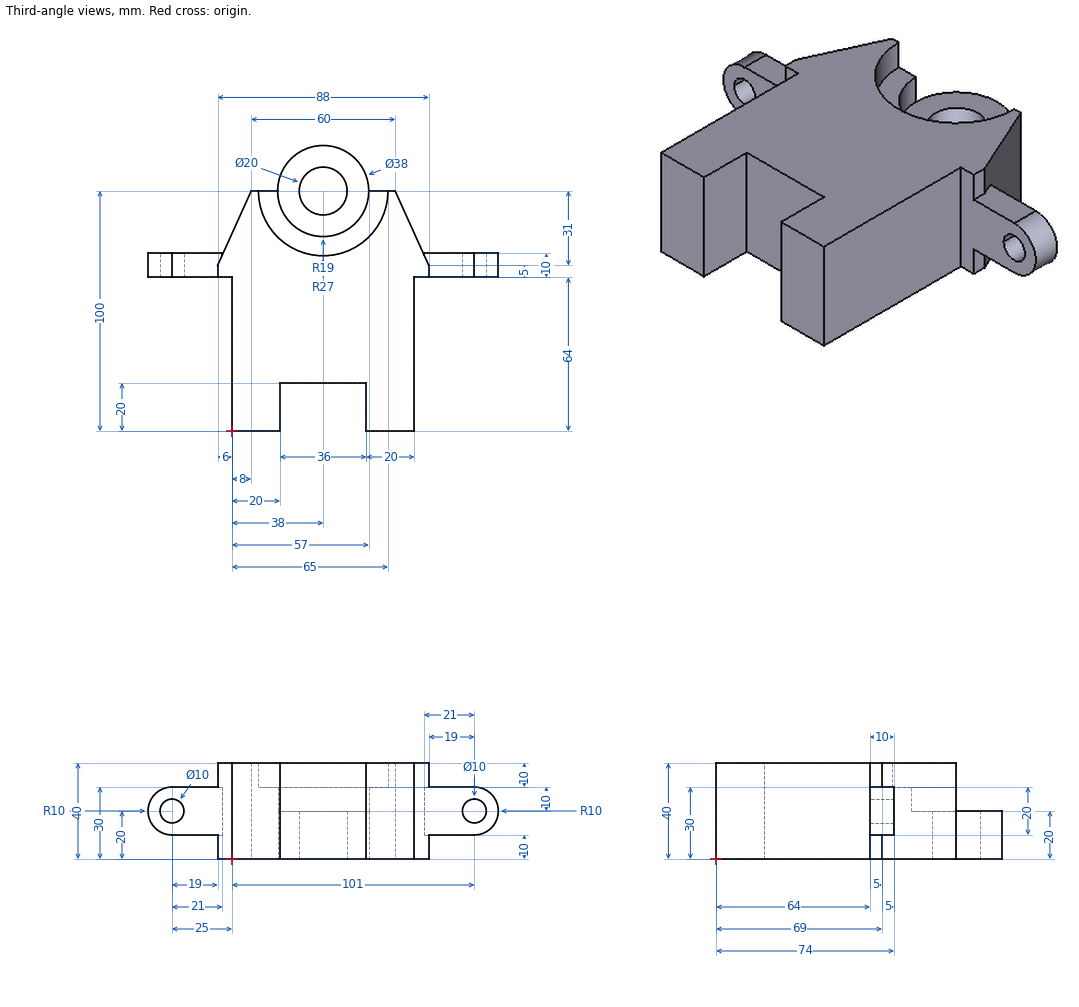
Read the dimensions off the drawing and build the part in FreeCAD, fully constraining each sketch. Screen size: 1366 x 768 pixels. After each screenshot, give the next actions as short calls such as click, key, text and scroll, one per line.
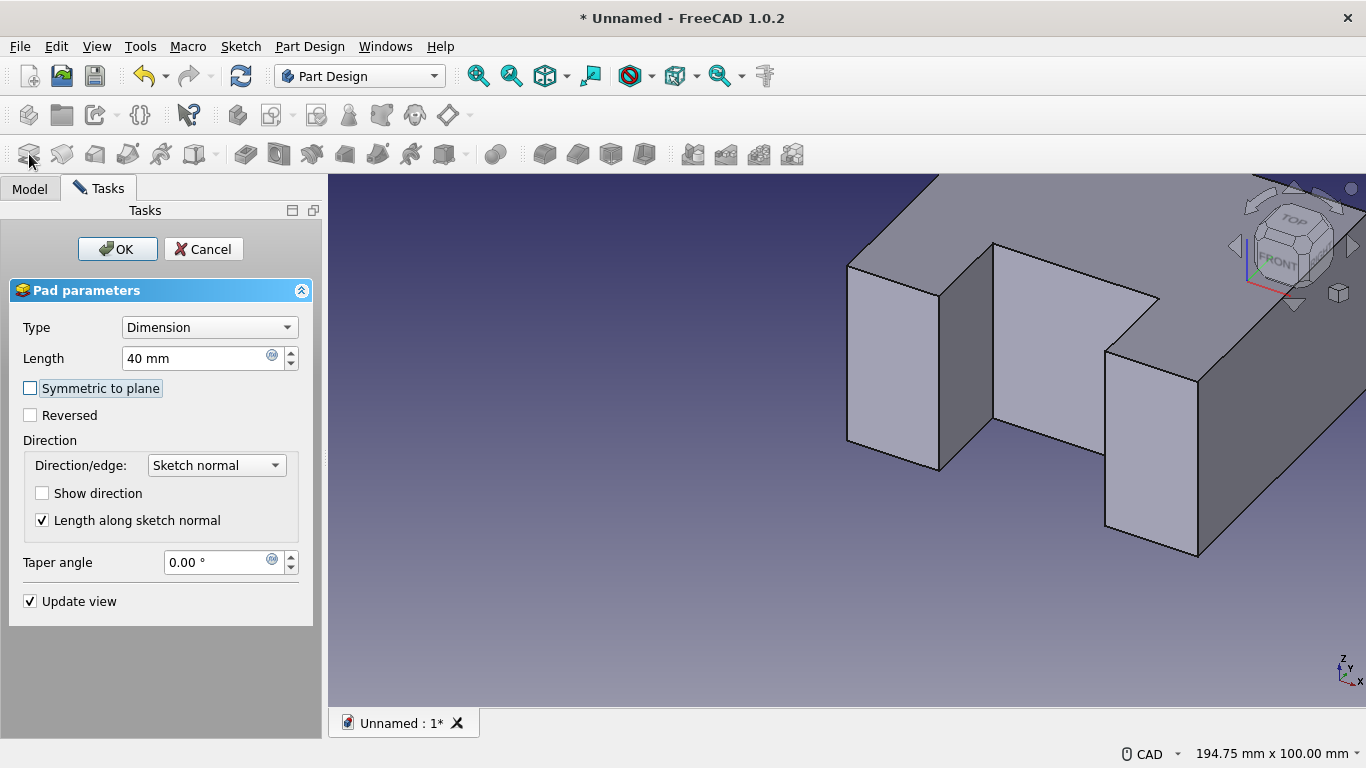
click(118, 249)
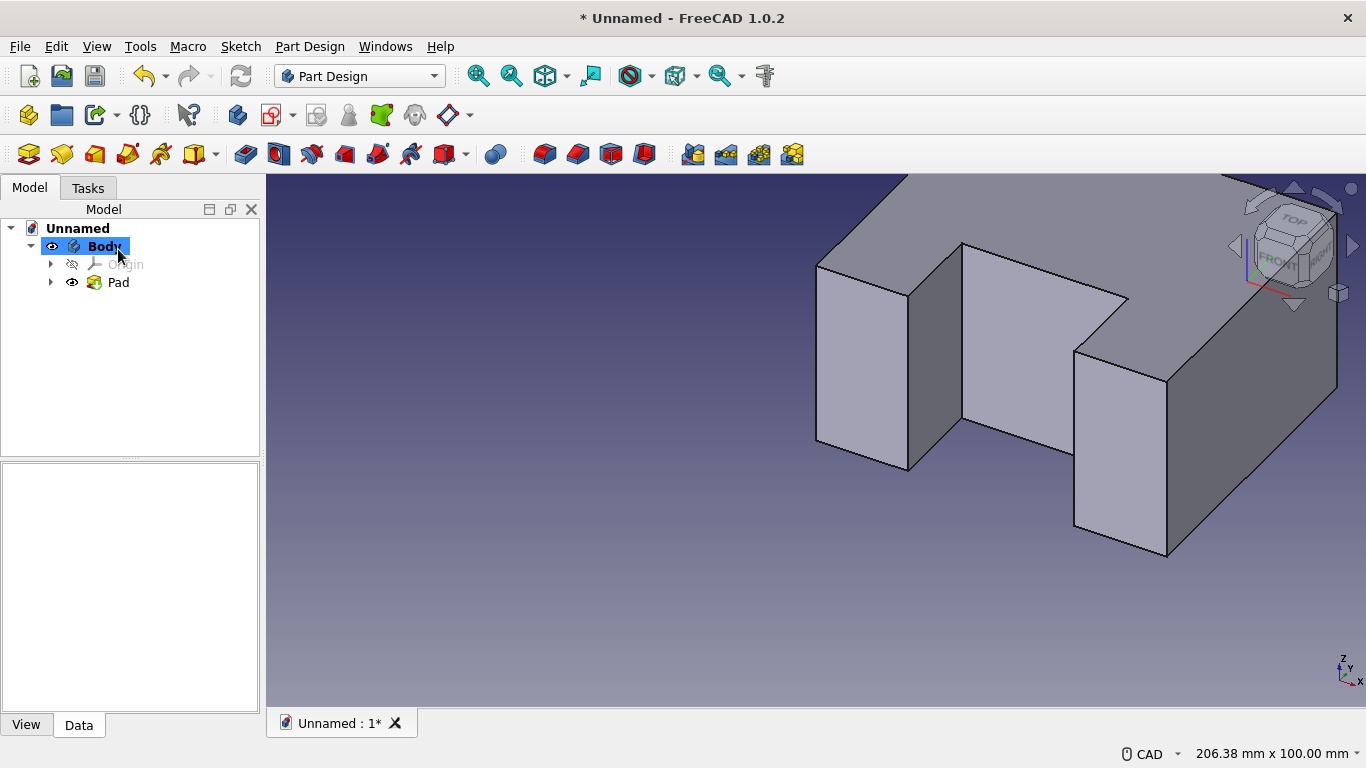
click(479, 76)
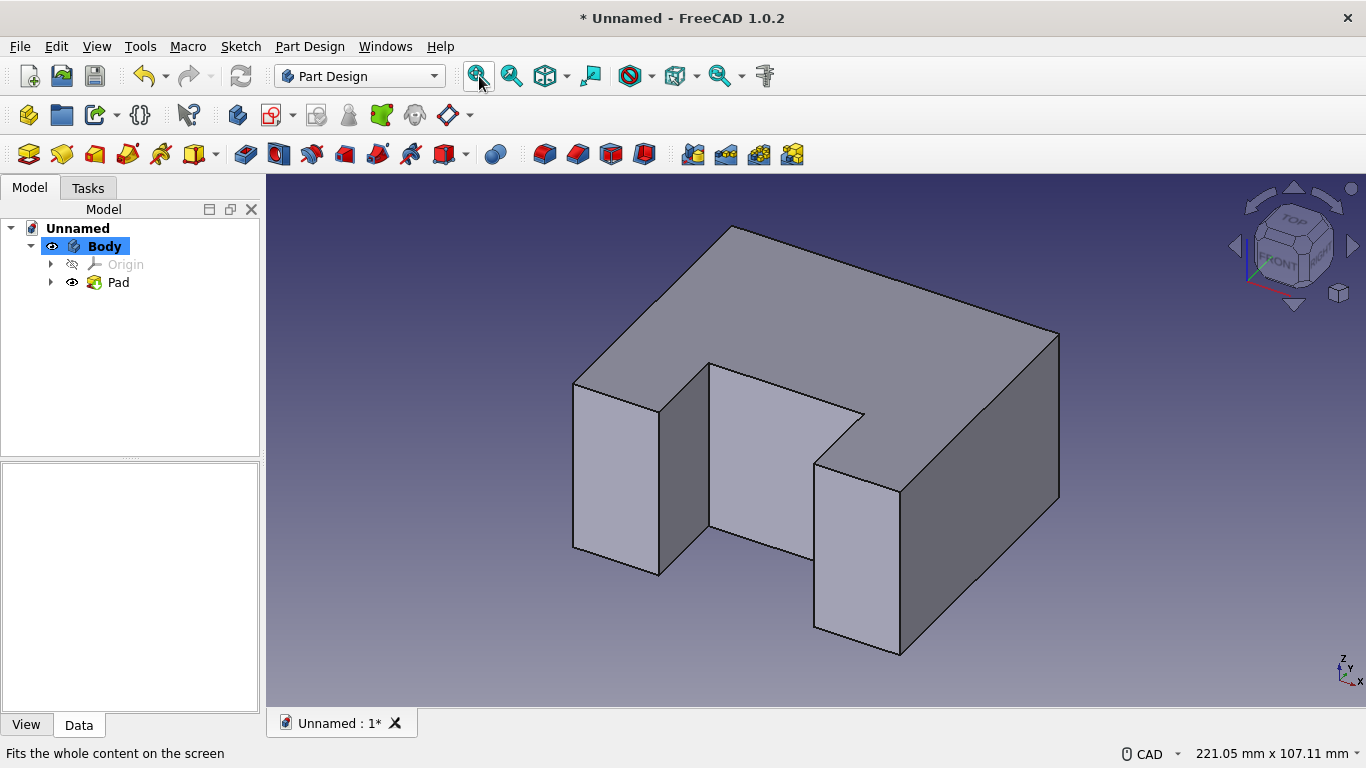
click(886, 351)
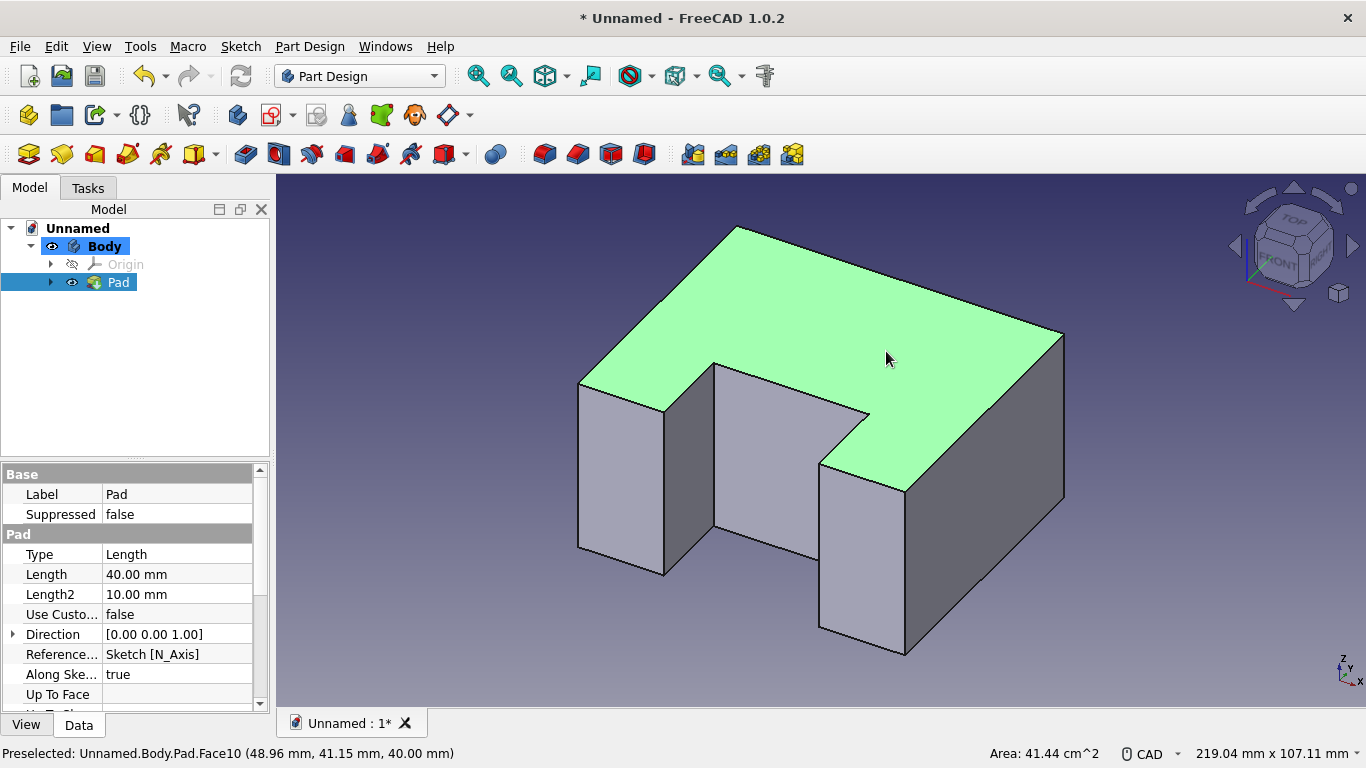
click(270, 116)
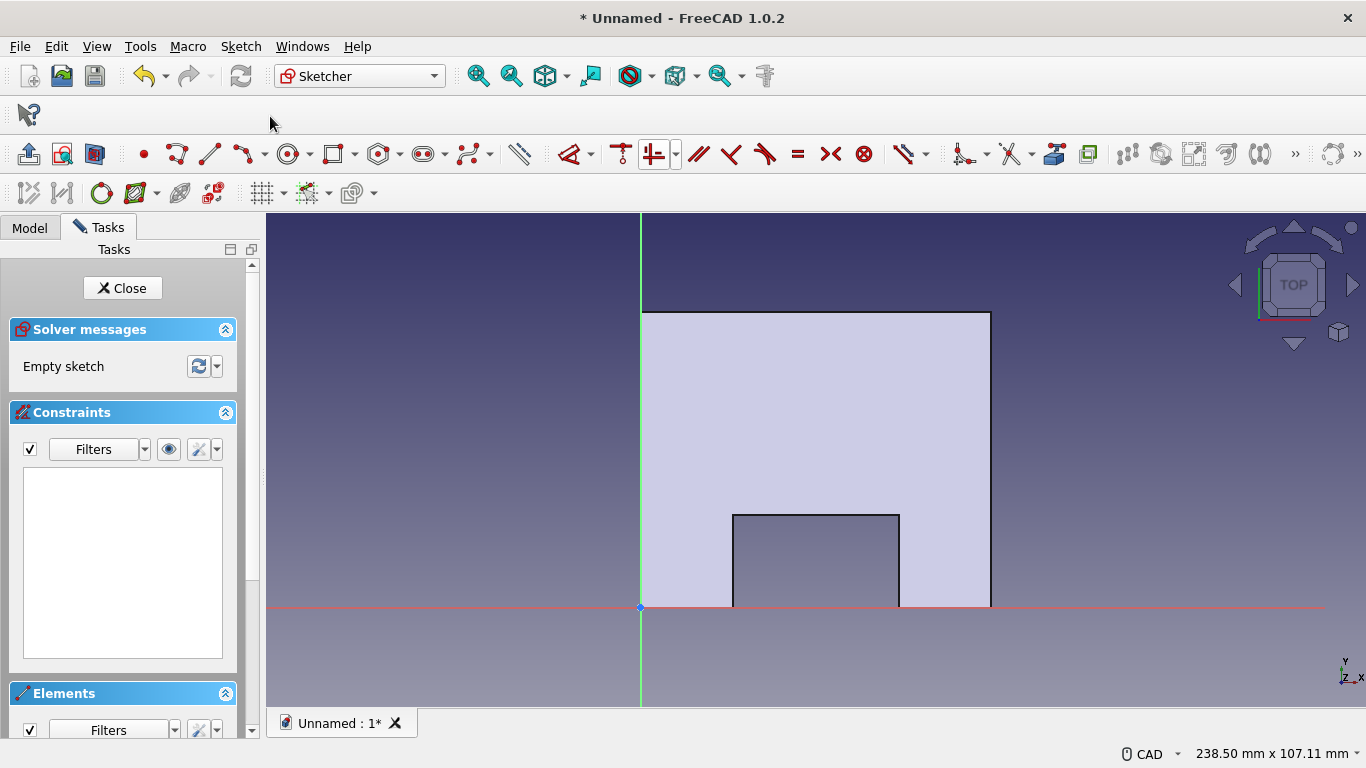
scroll(608, 629, down, 2)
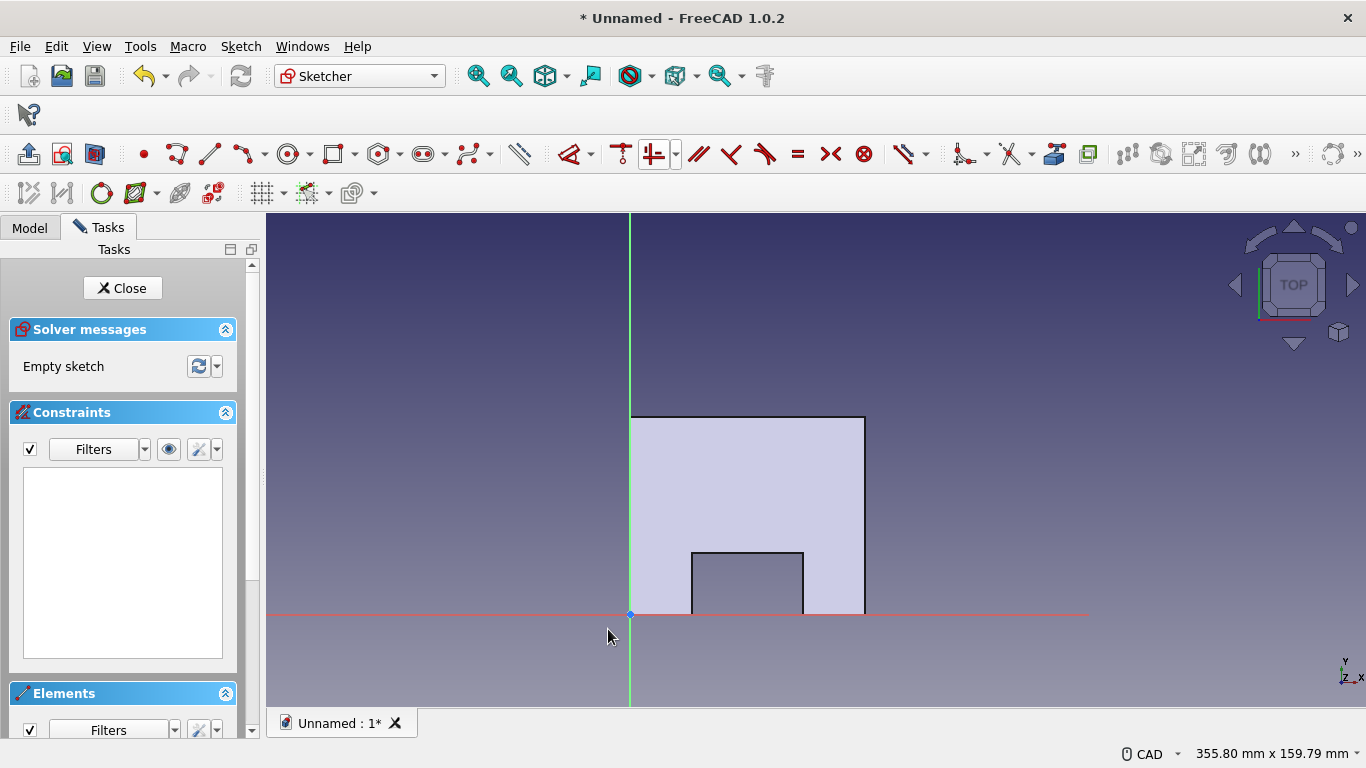
click(177, 154)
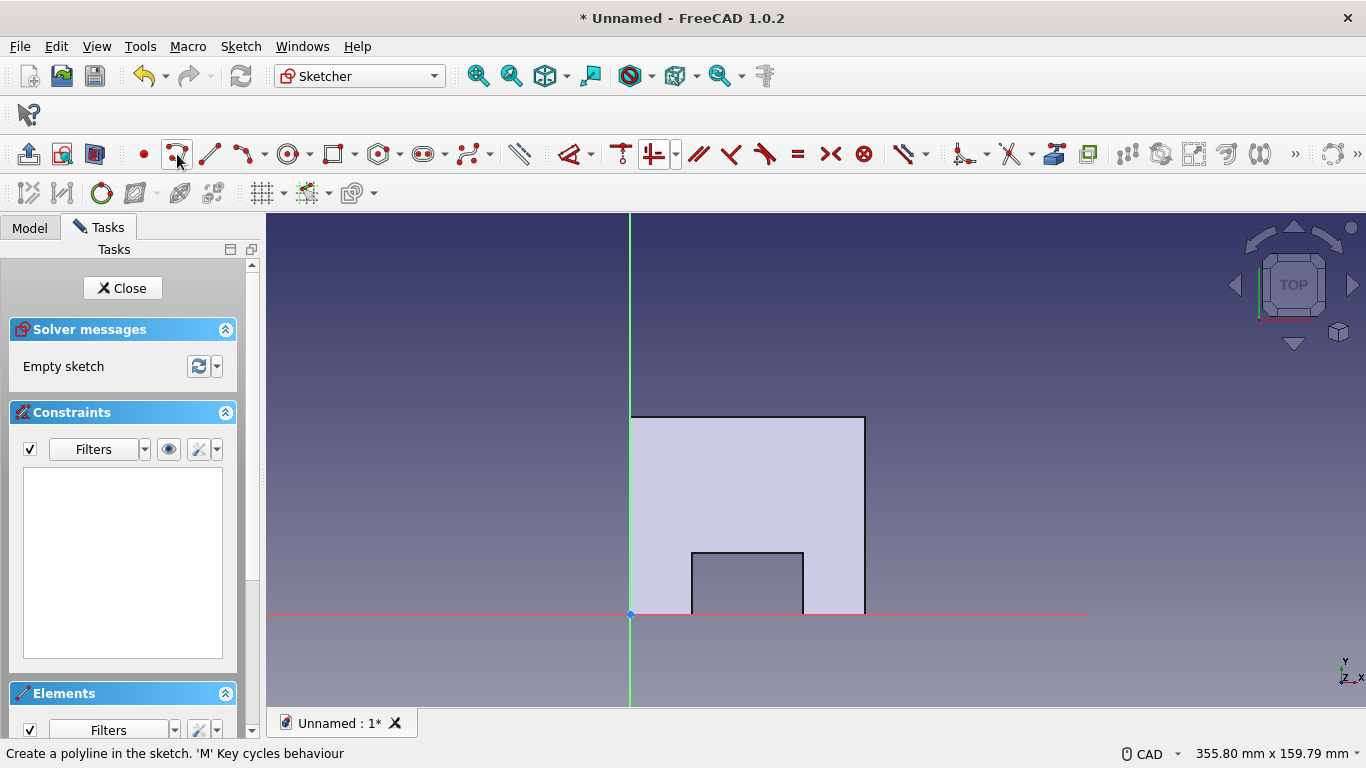
click(611, 417)
click(884, 417)
click(884, 402)
click(840, 306)
click(655, 306)
click(611, 402)
click(611, 418)
key(Escape)
key(Escape)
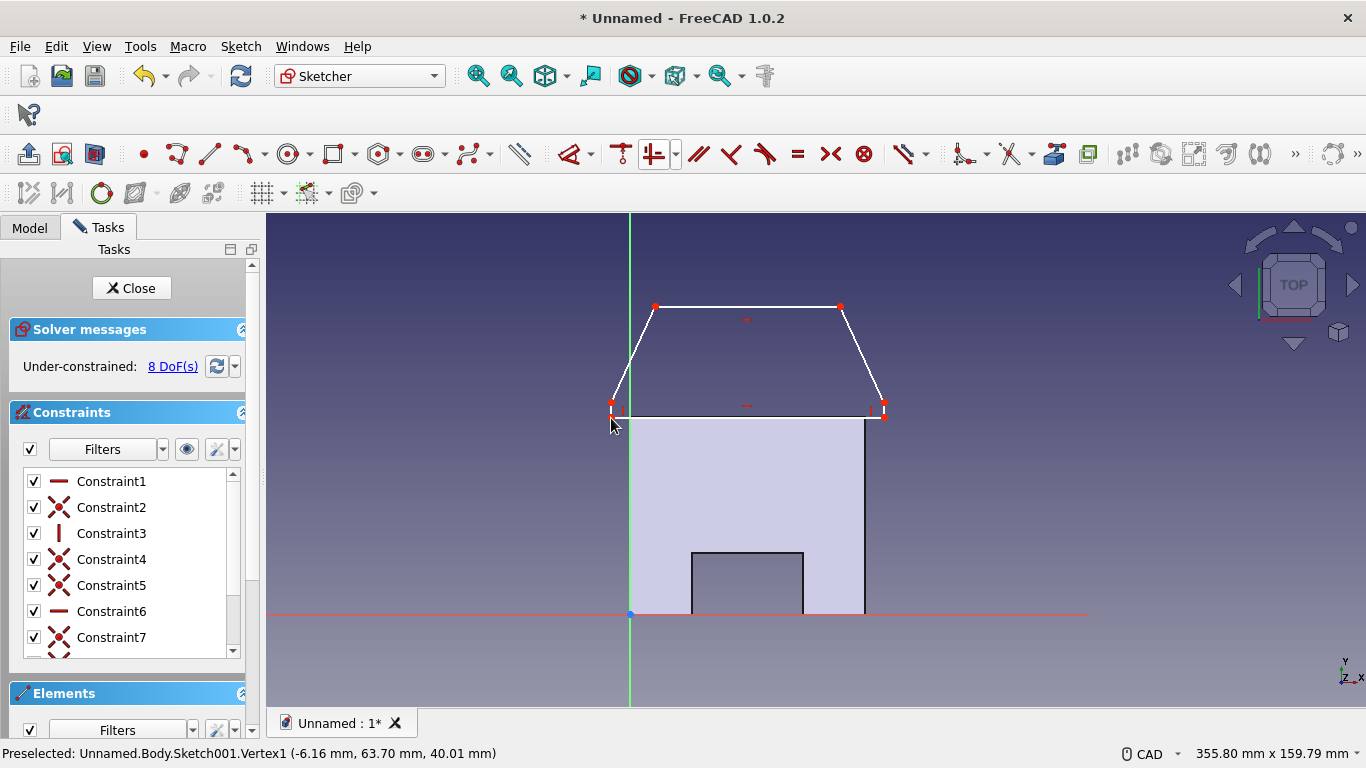
click(568, 154)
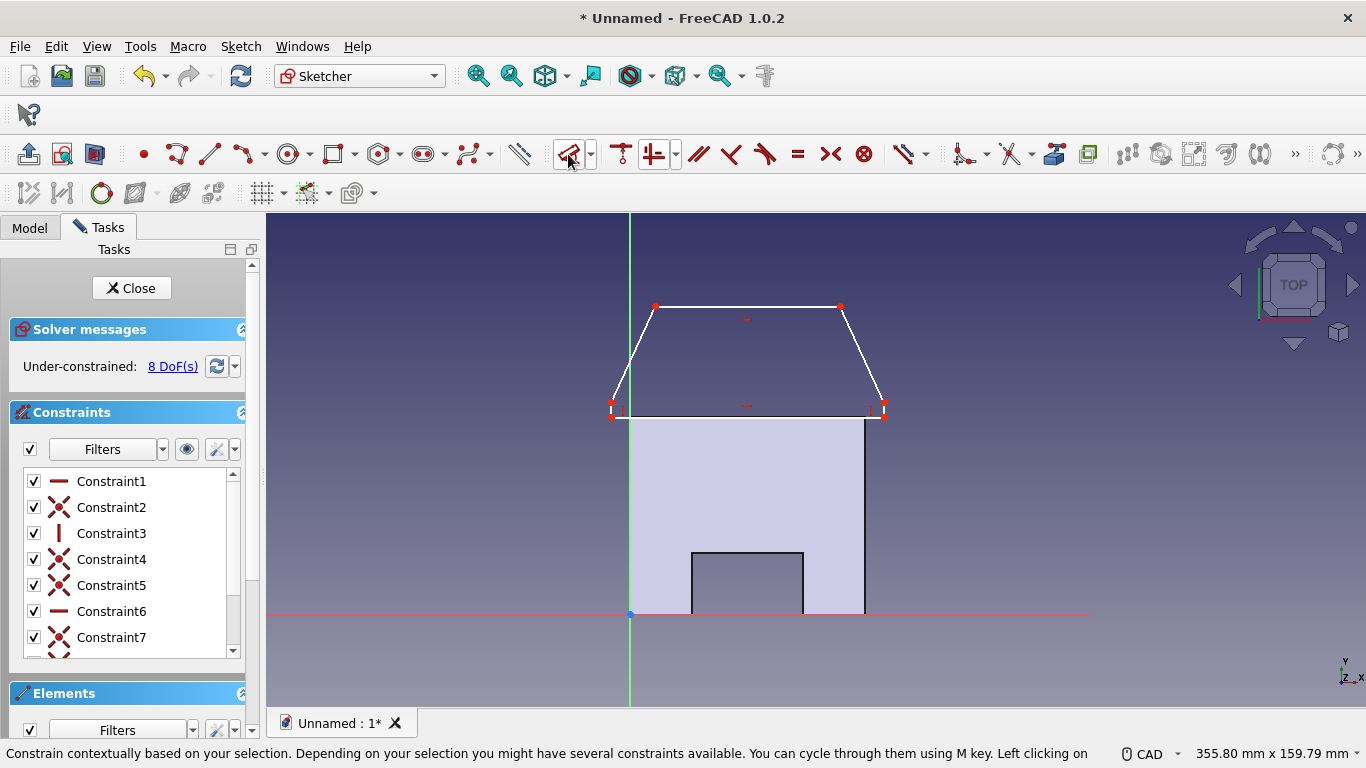
scroll(884, 410, up, 5)